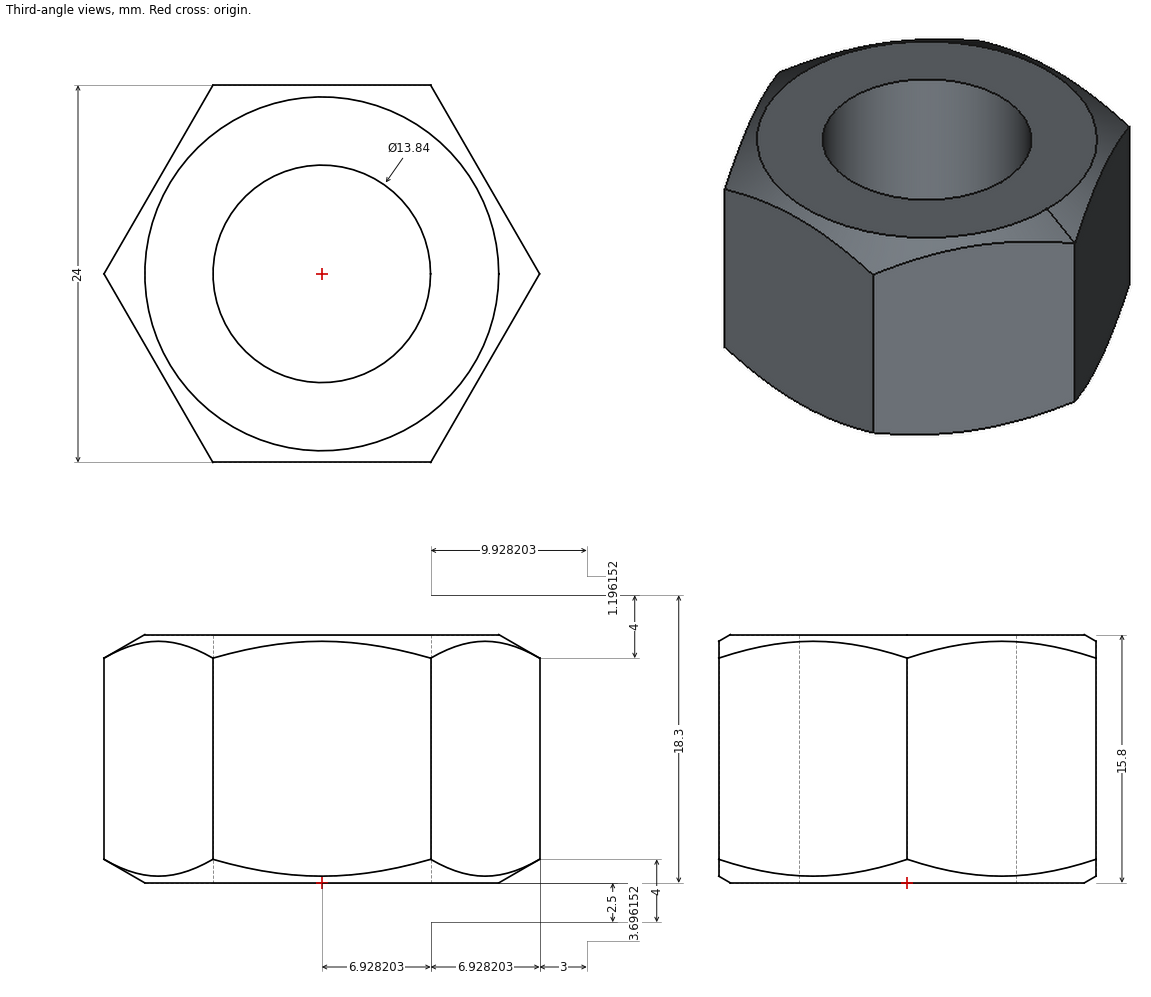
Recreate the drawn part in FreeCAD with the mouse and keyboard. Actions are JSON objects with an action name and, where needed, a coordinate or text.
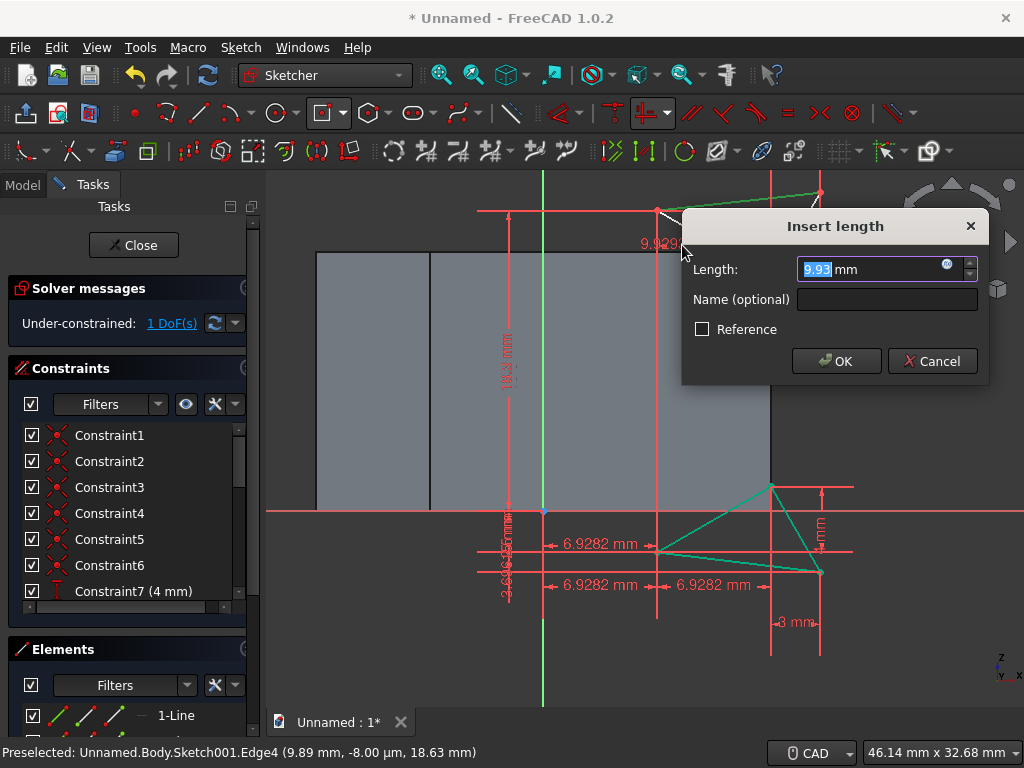
{"action": "type", "text": "9.928203"}
{"action": "key", "text": "Return"}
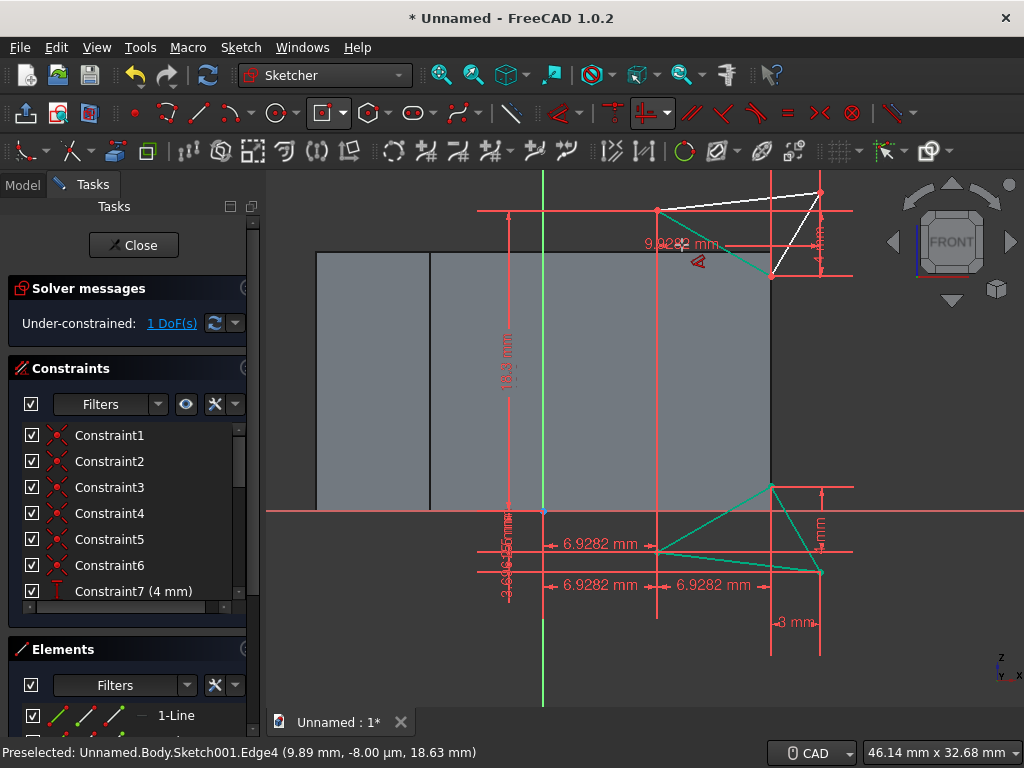
{"action": "scroll", "coordinate": [706, 205], "scroll_direction": "up", "scroll_amount": 4}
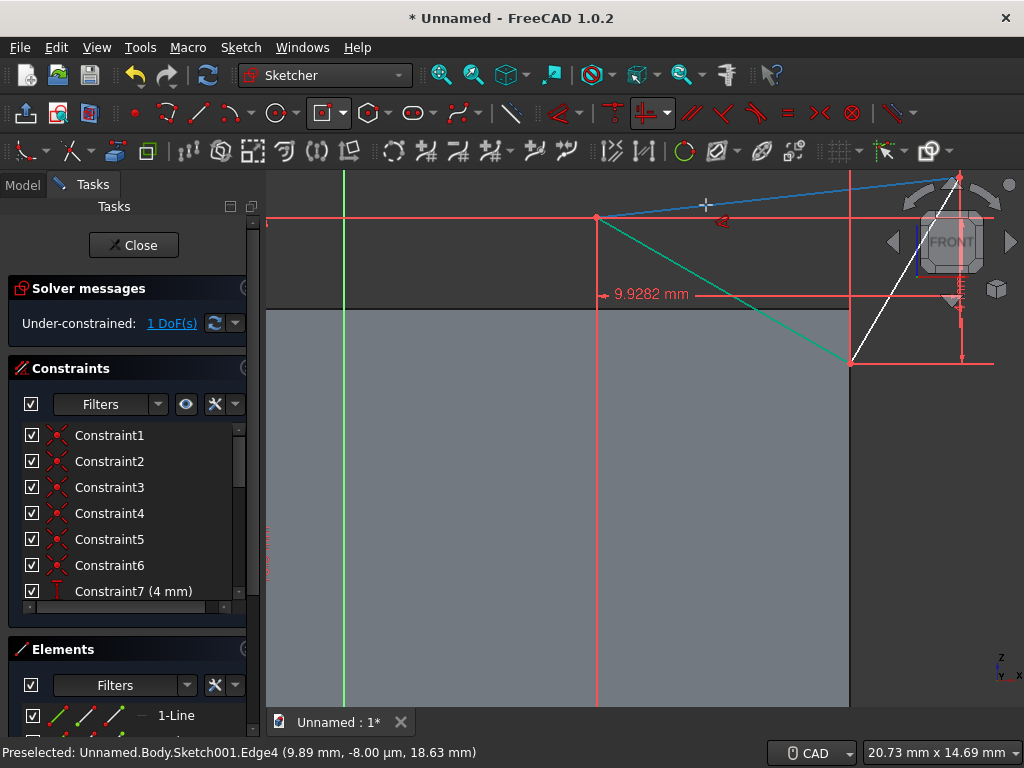
{"action": "left_click", "coordinate": [706, 206]}
{"action": "left_click", "coordinate": [563, 208]}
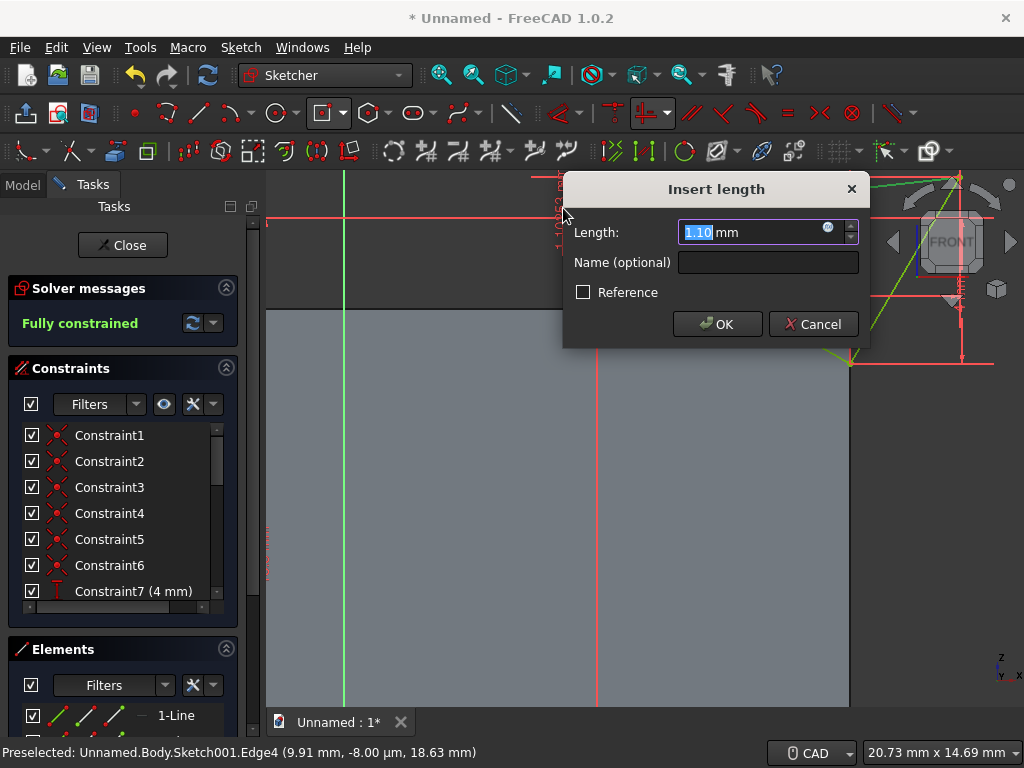
{"action": "type", "text": "1.196152"}
{"action": "key", "text": "Return"}
{"action": "key", "text": "Escape"}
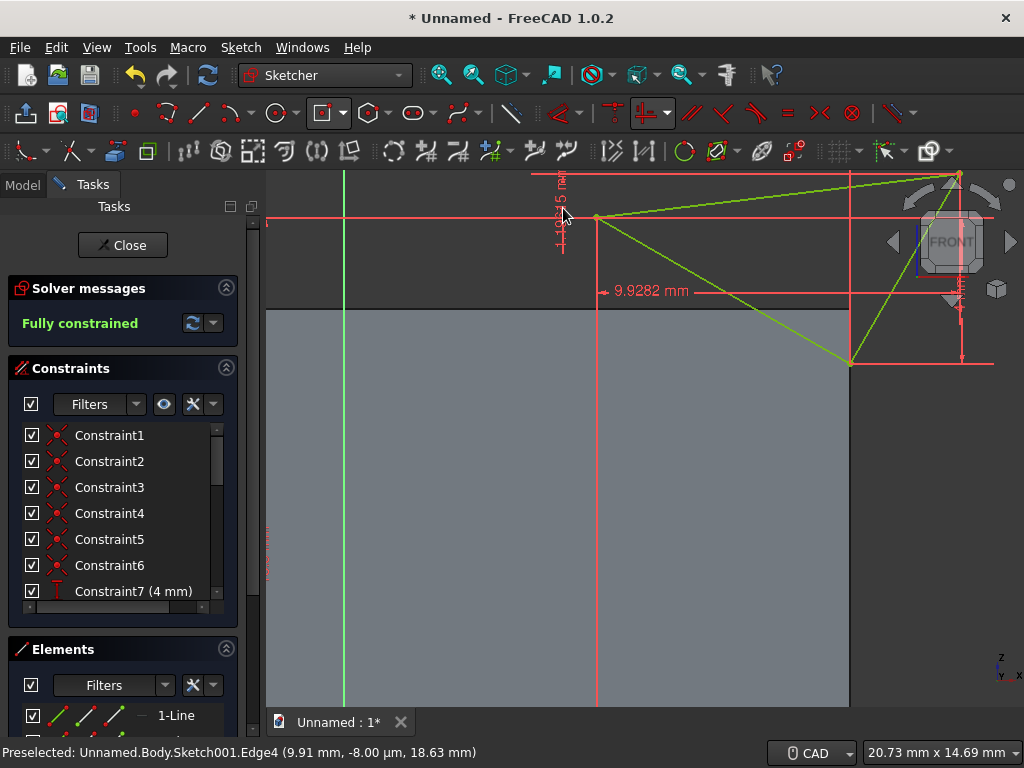
{"action": "left_click", "coordinate": [123, 245]}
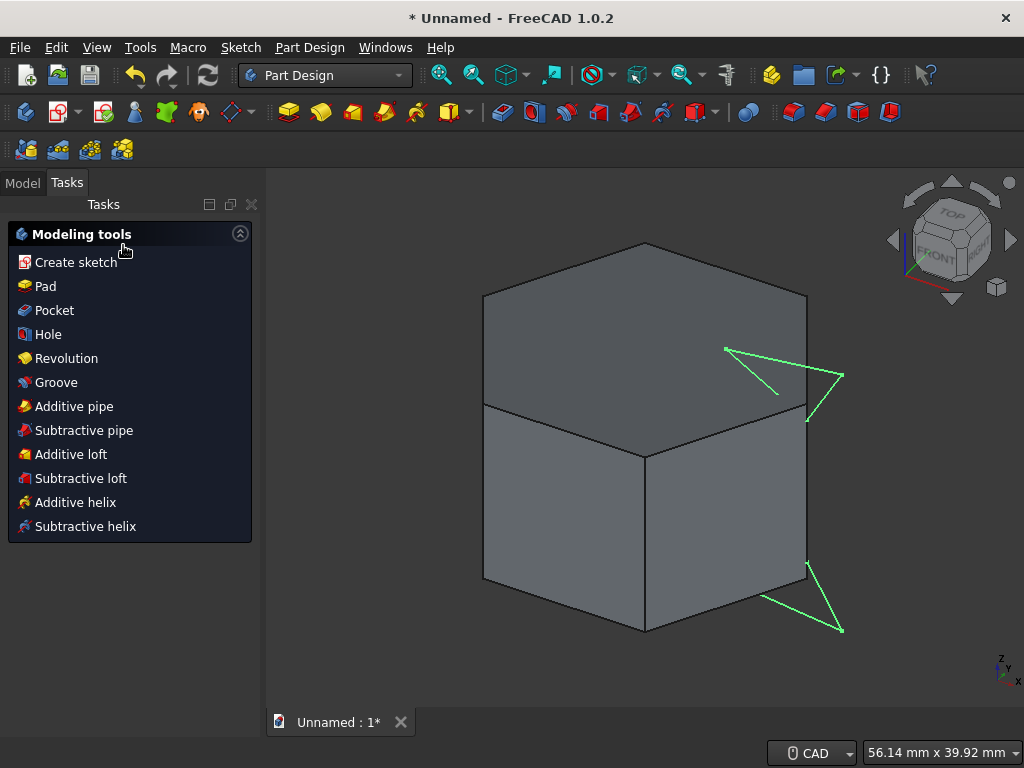
{"action": "left_click", "coordinate": [568, 112]}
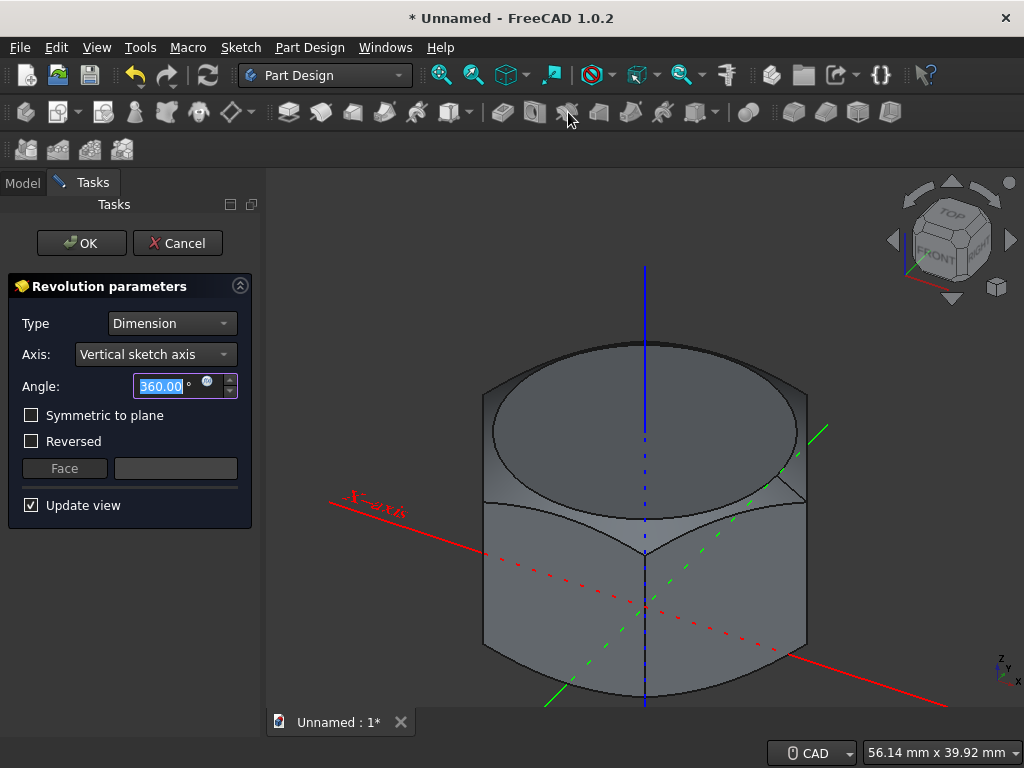
{"action": "left_click", "coordinate": [82, 243]}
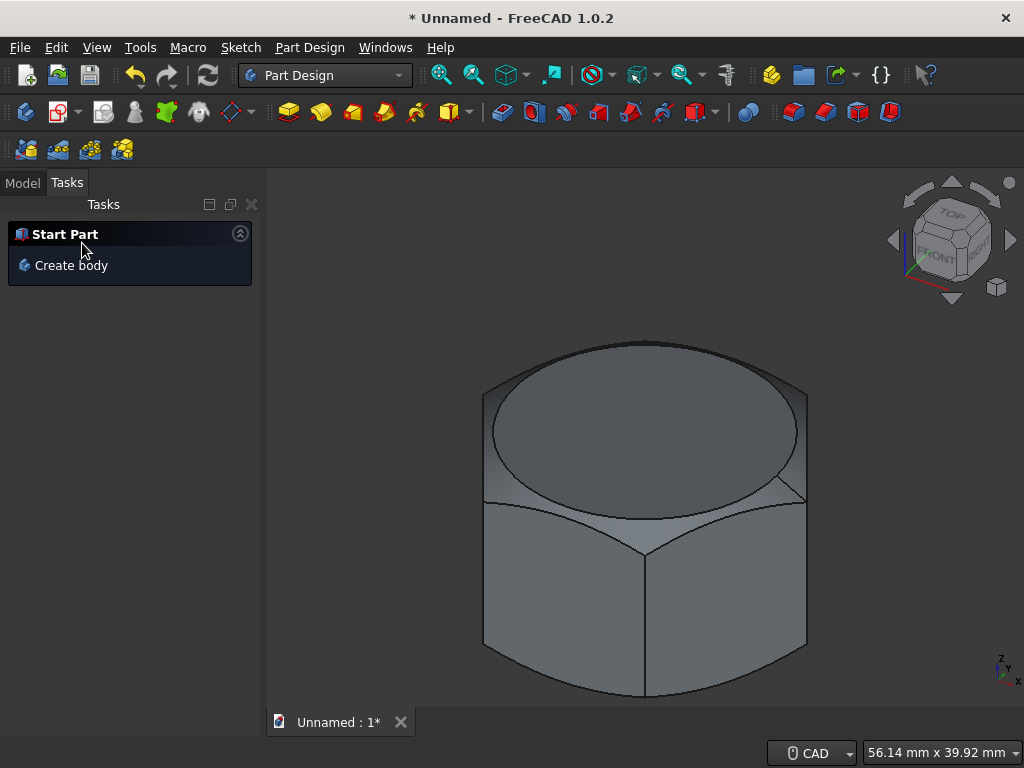
{"action": "left_click", "coordinate": [442, 76]}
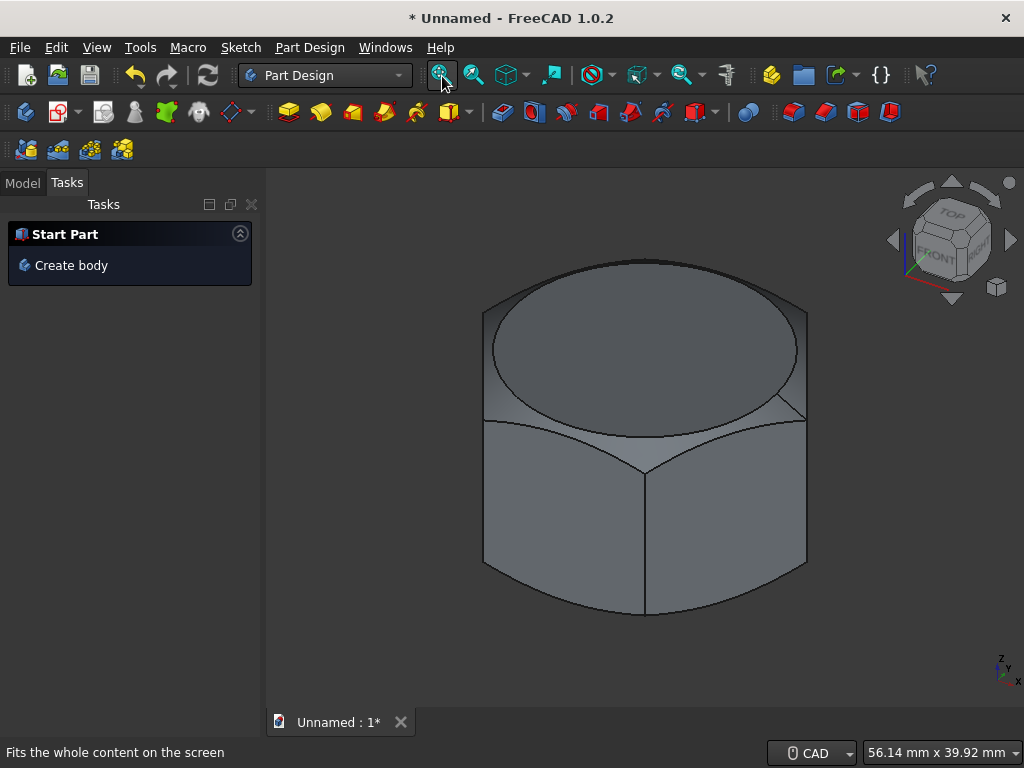
{"action": "key", "text": "5"}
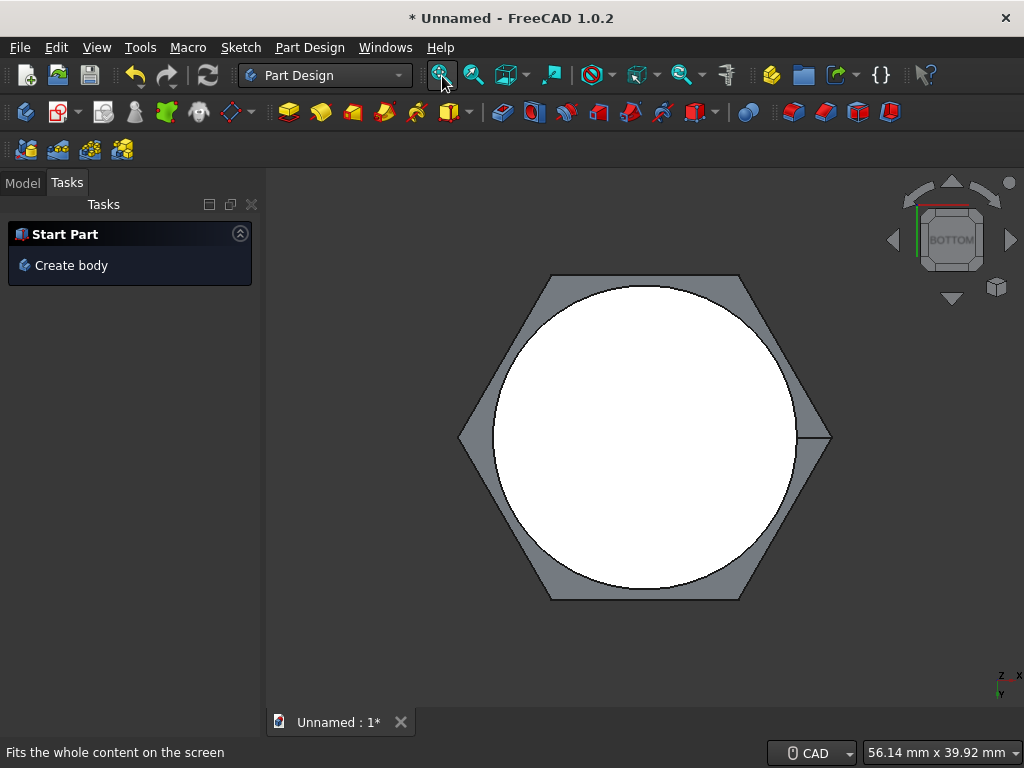
{"action": "left_click", "coordinate": [645, 436]}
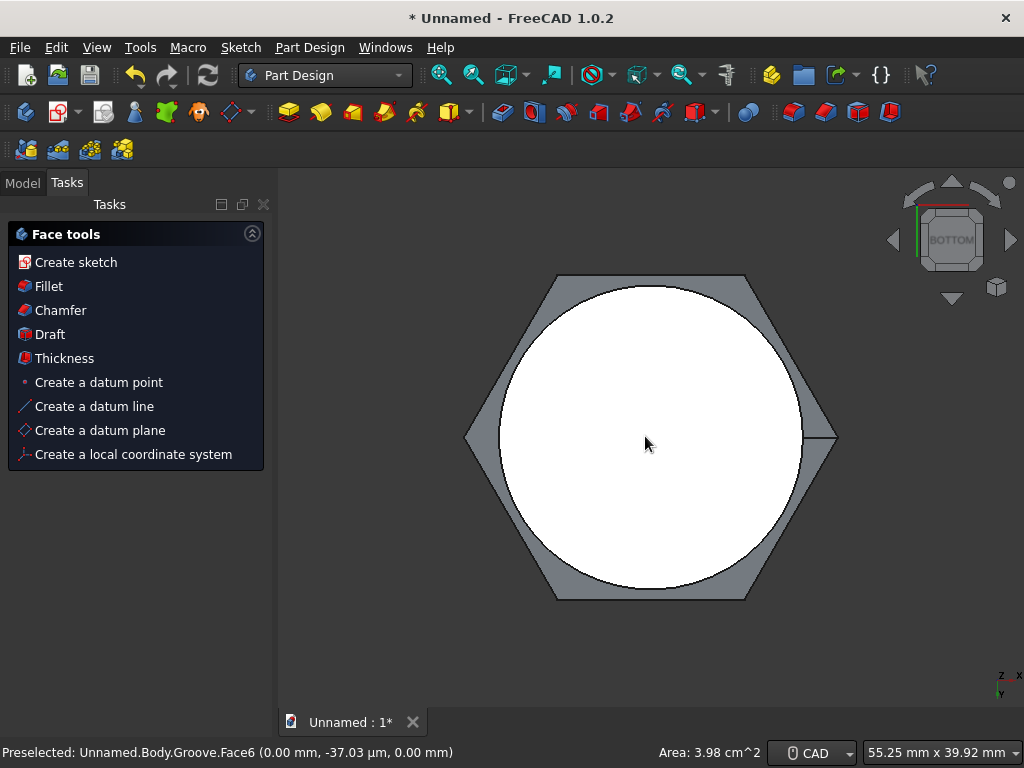
{"action": "left_click", "coordinate": [58, 112]}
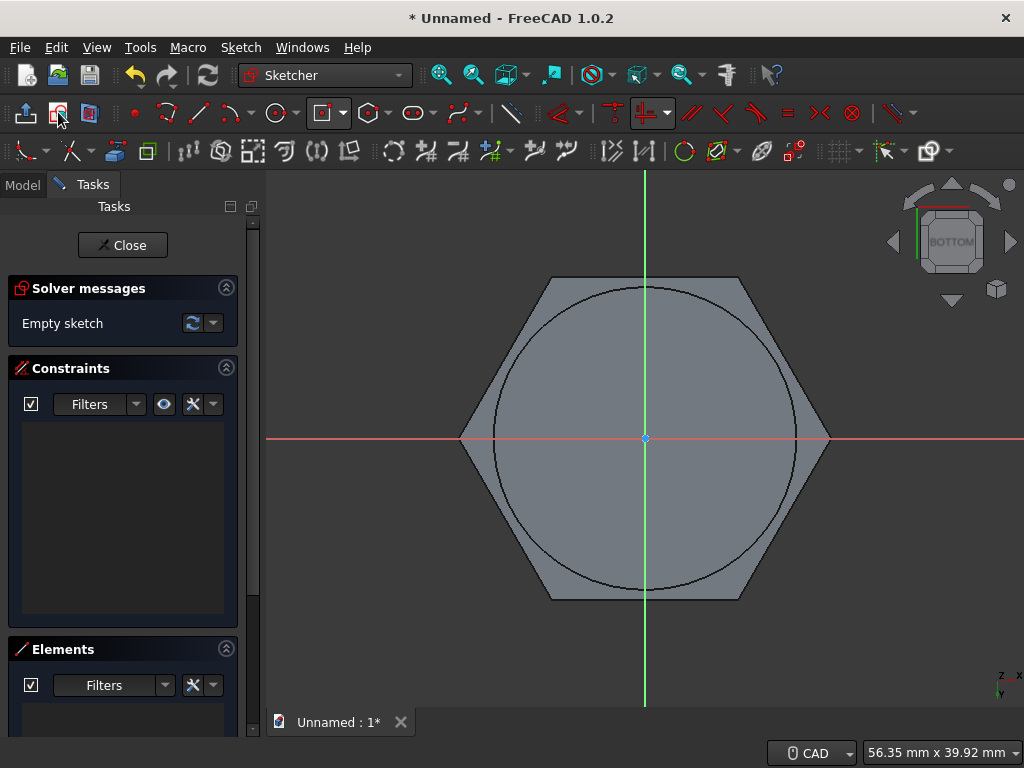
{"action": "scroll", "coordinate": [728, 438], "scroll_direction": "up", "scroll_amount": 3}